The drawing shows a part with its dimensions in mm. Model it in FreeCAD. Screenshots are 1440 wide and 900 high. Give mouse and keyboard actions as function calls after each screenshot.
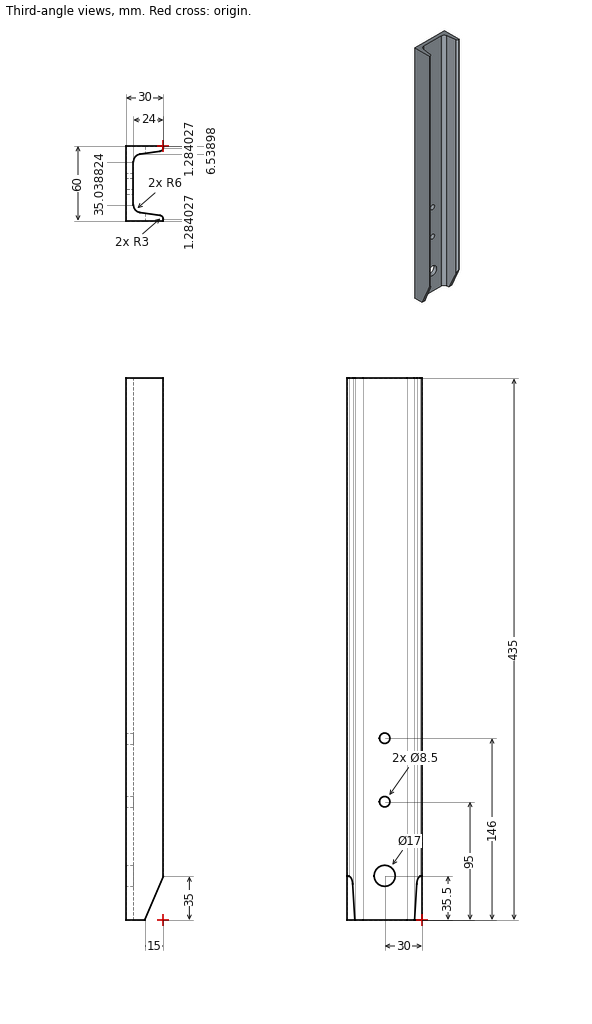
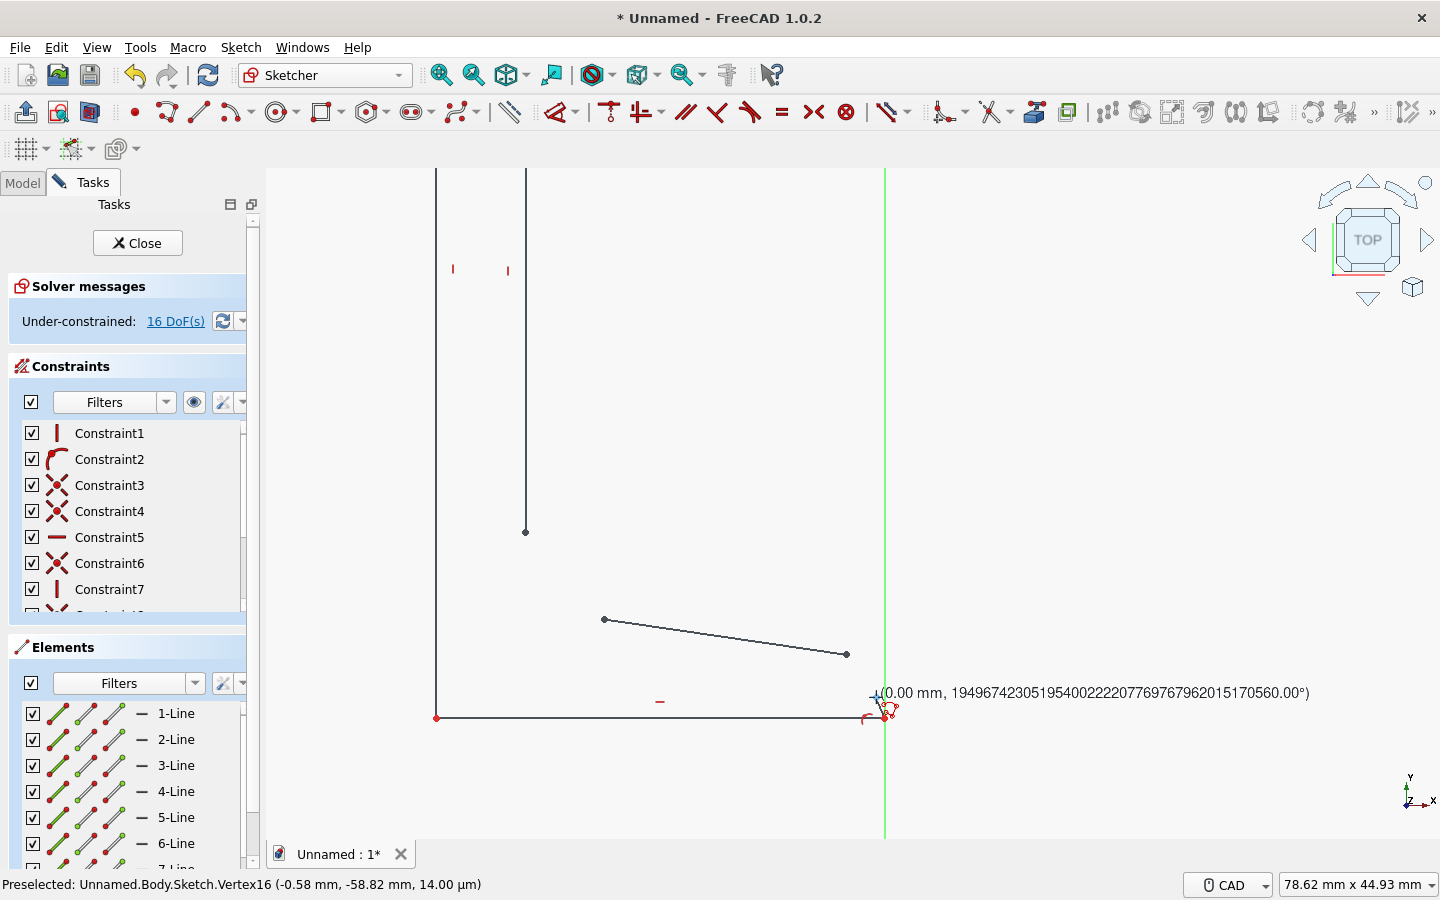
key(g)
key(3)
key(a)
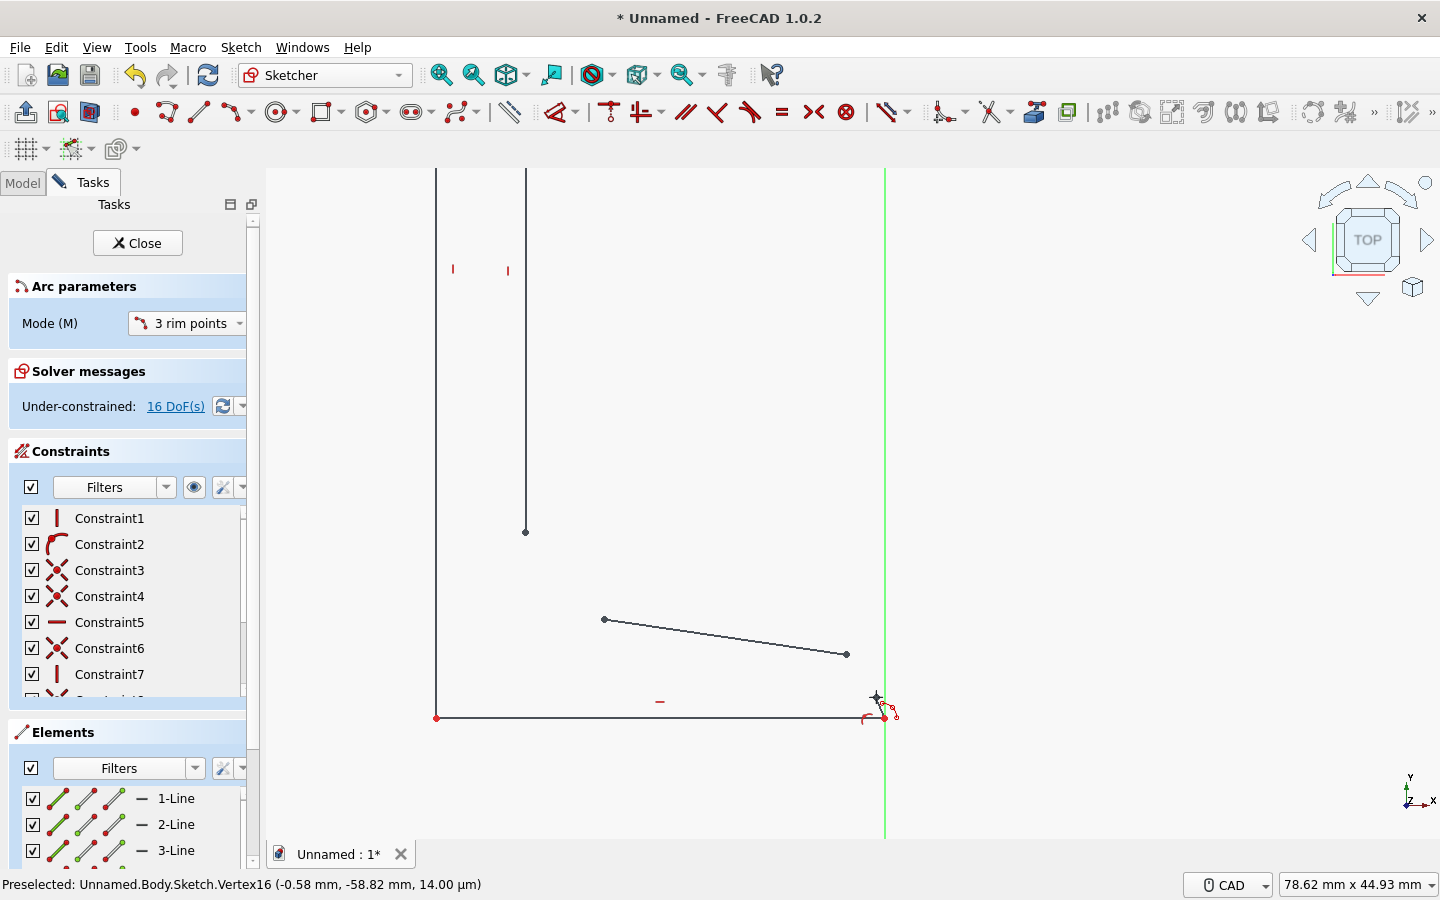
click(605, 619)
click(526, 533)
click(548, 588)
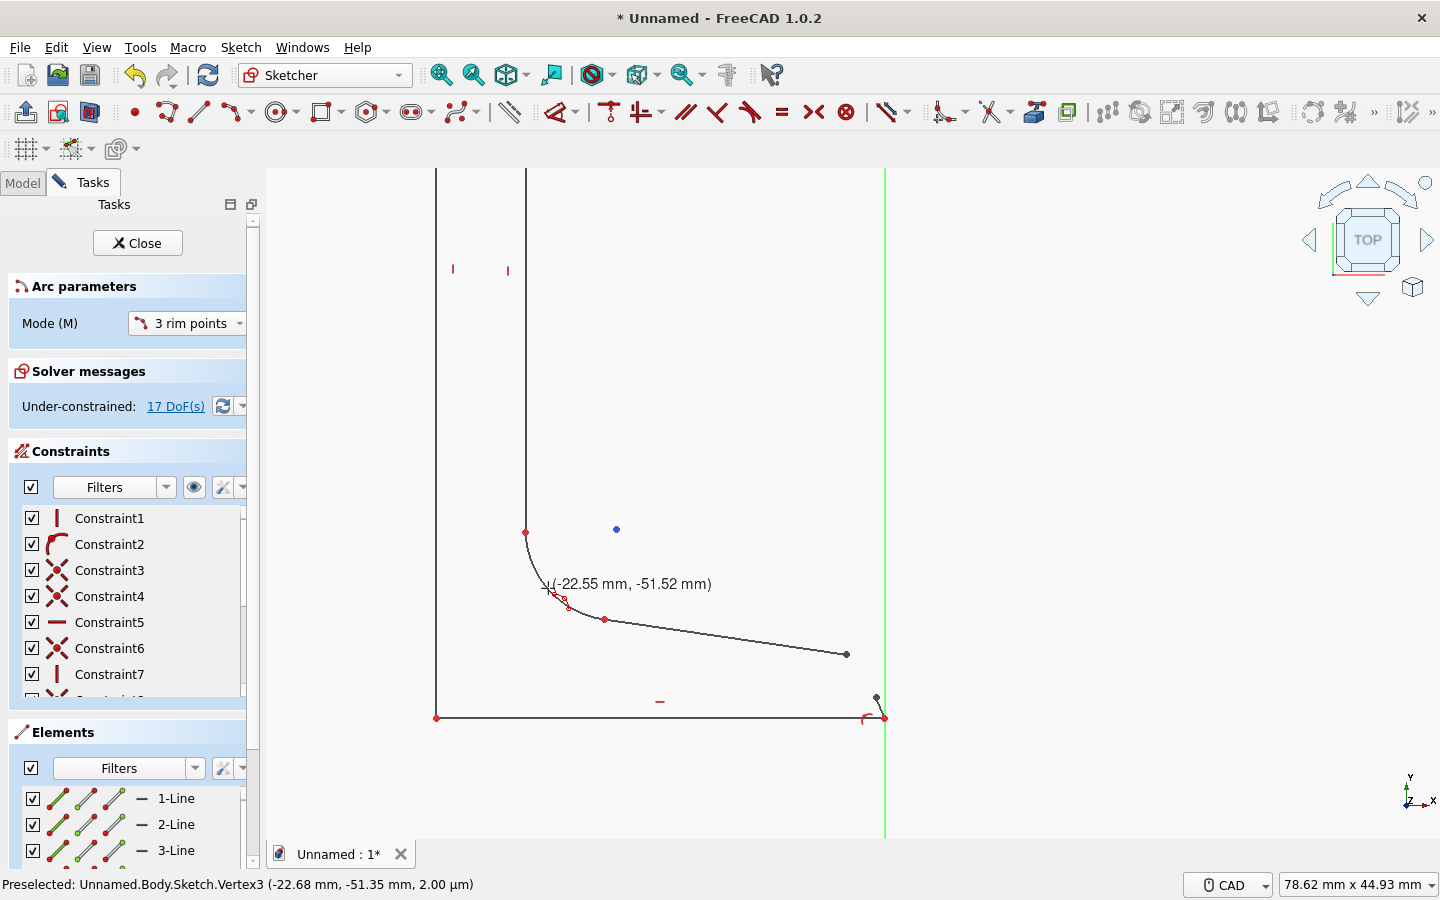
scroll(886, 696, down, 4)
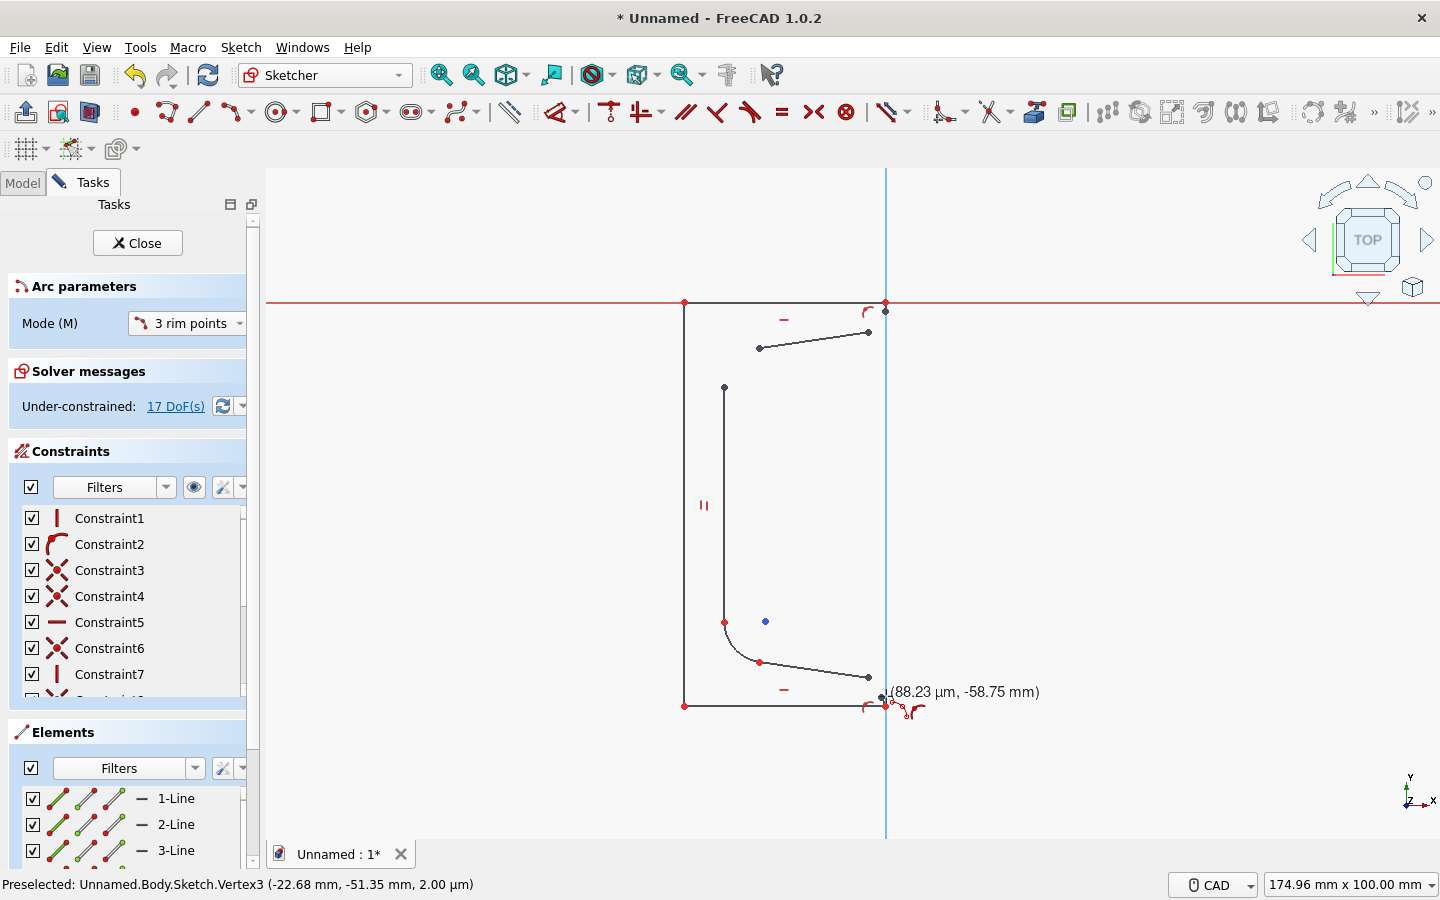
click(724, 387)
click(760, 348)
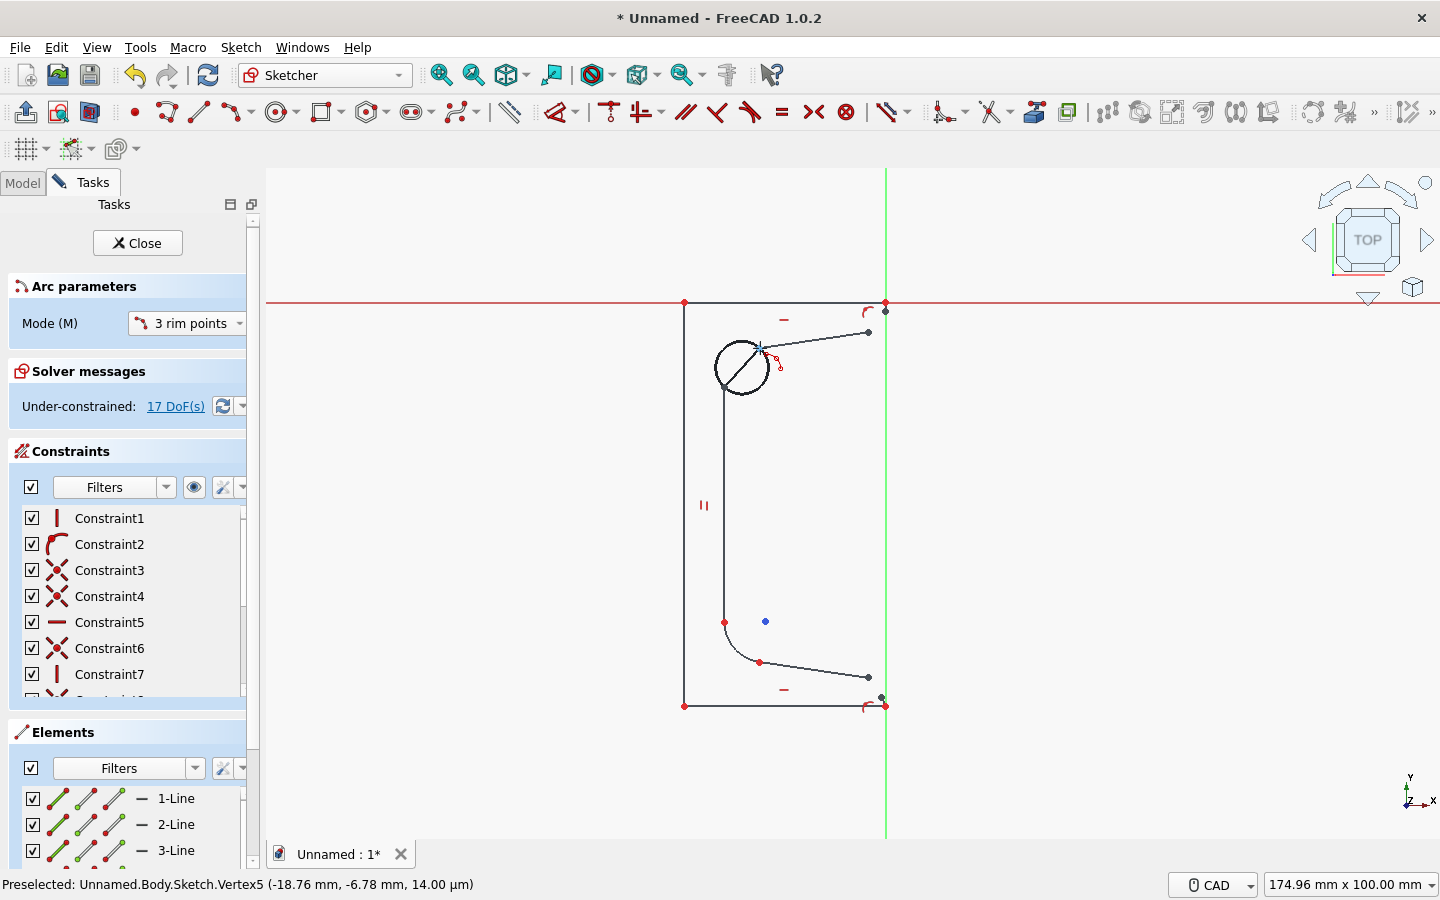
scroll(735, 360, up, 3)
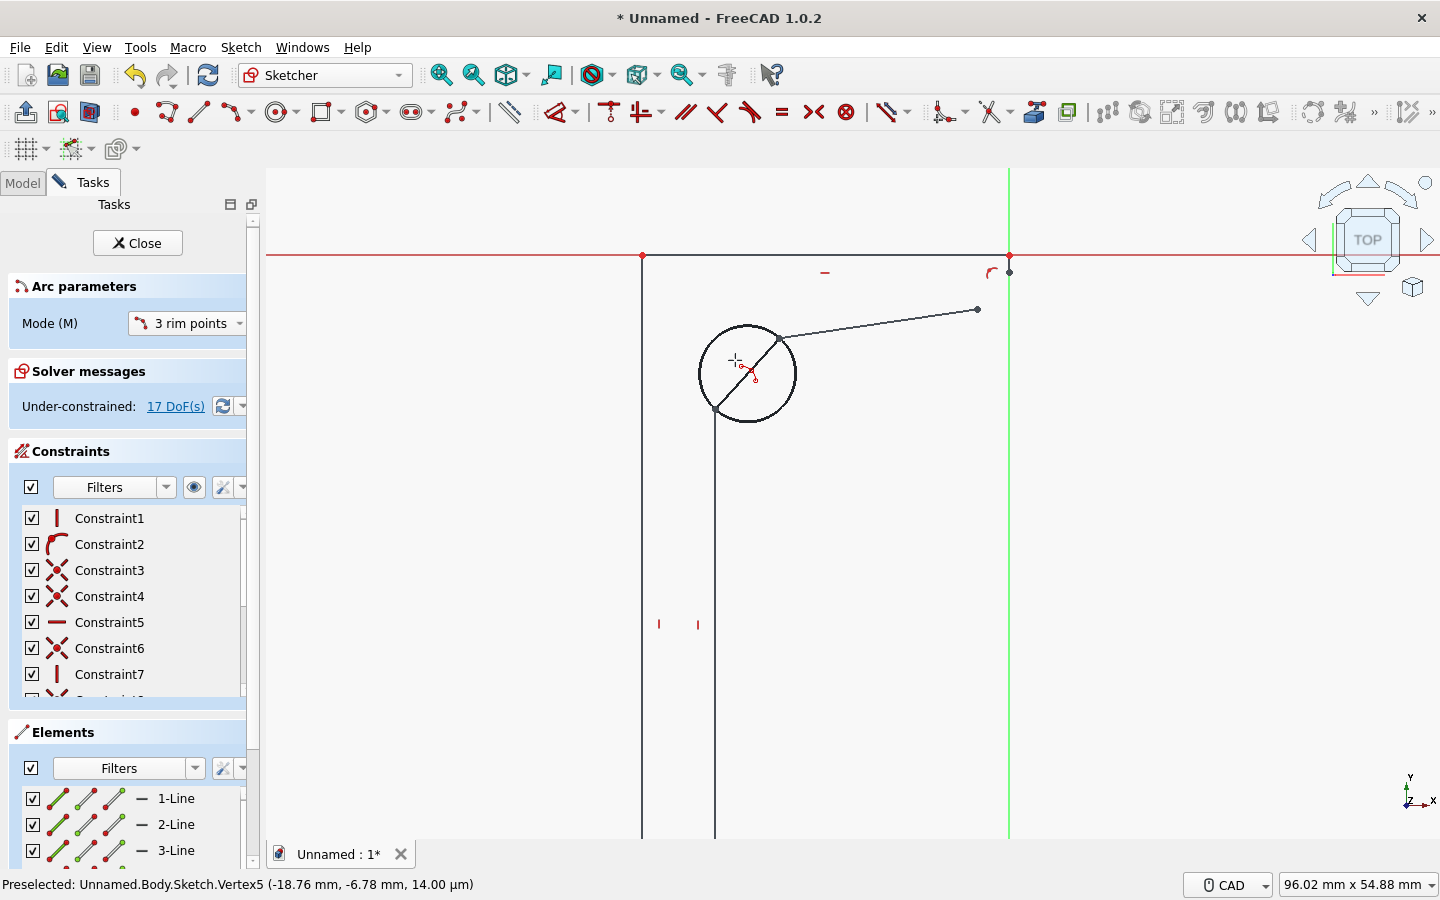
click(734, 360)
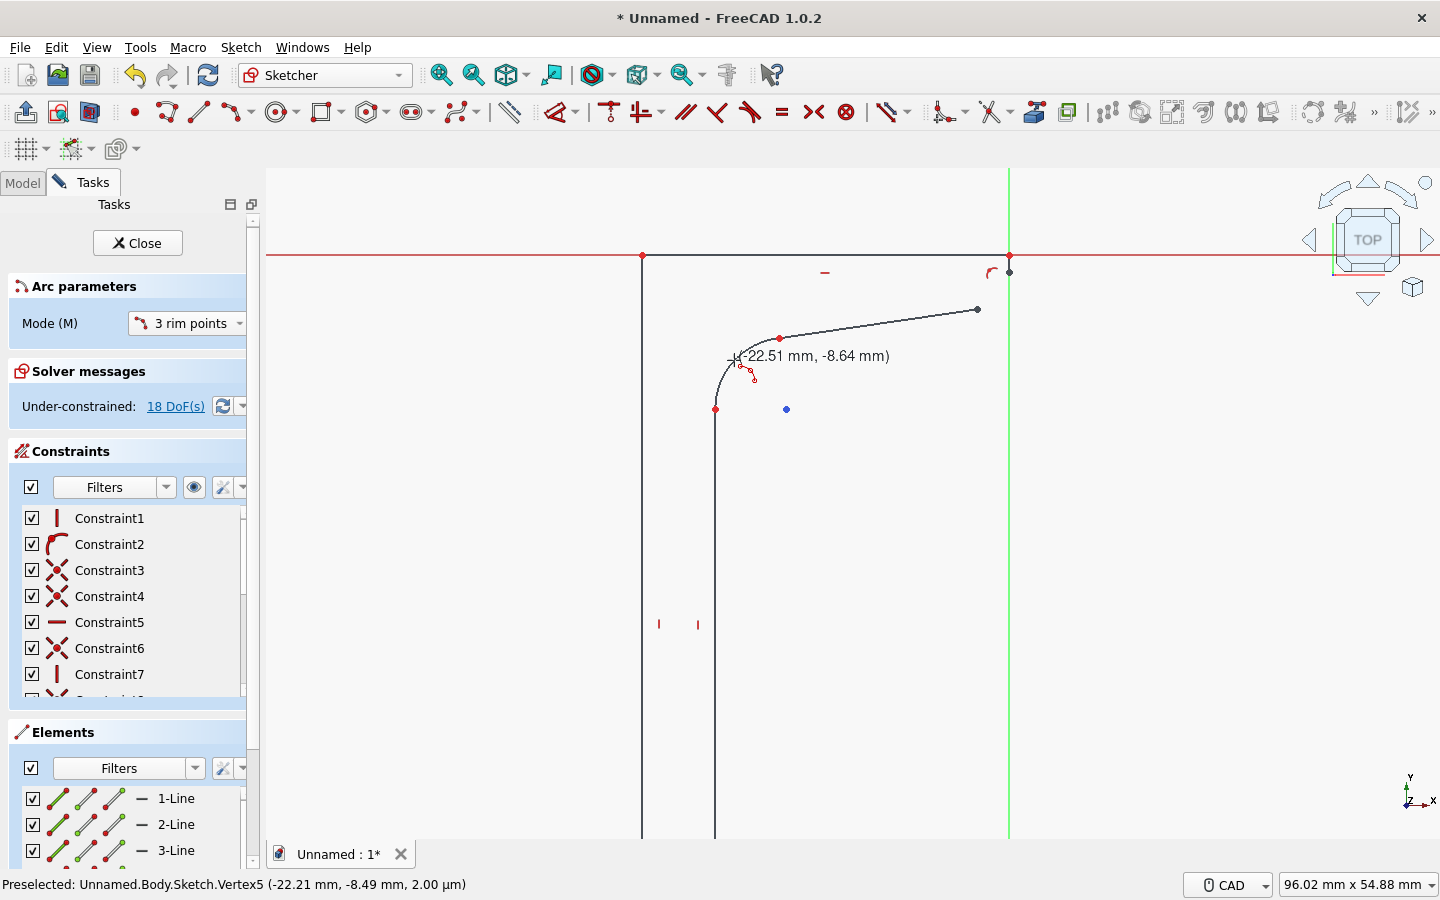
click(978, 309)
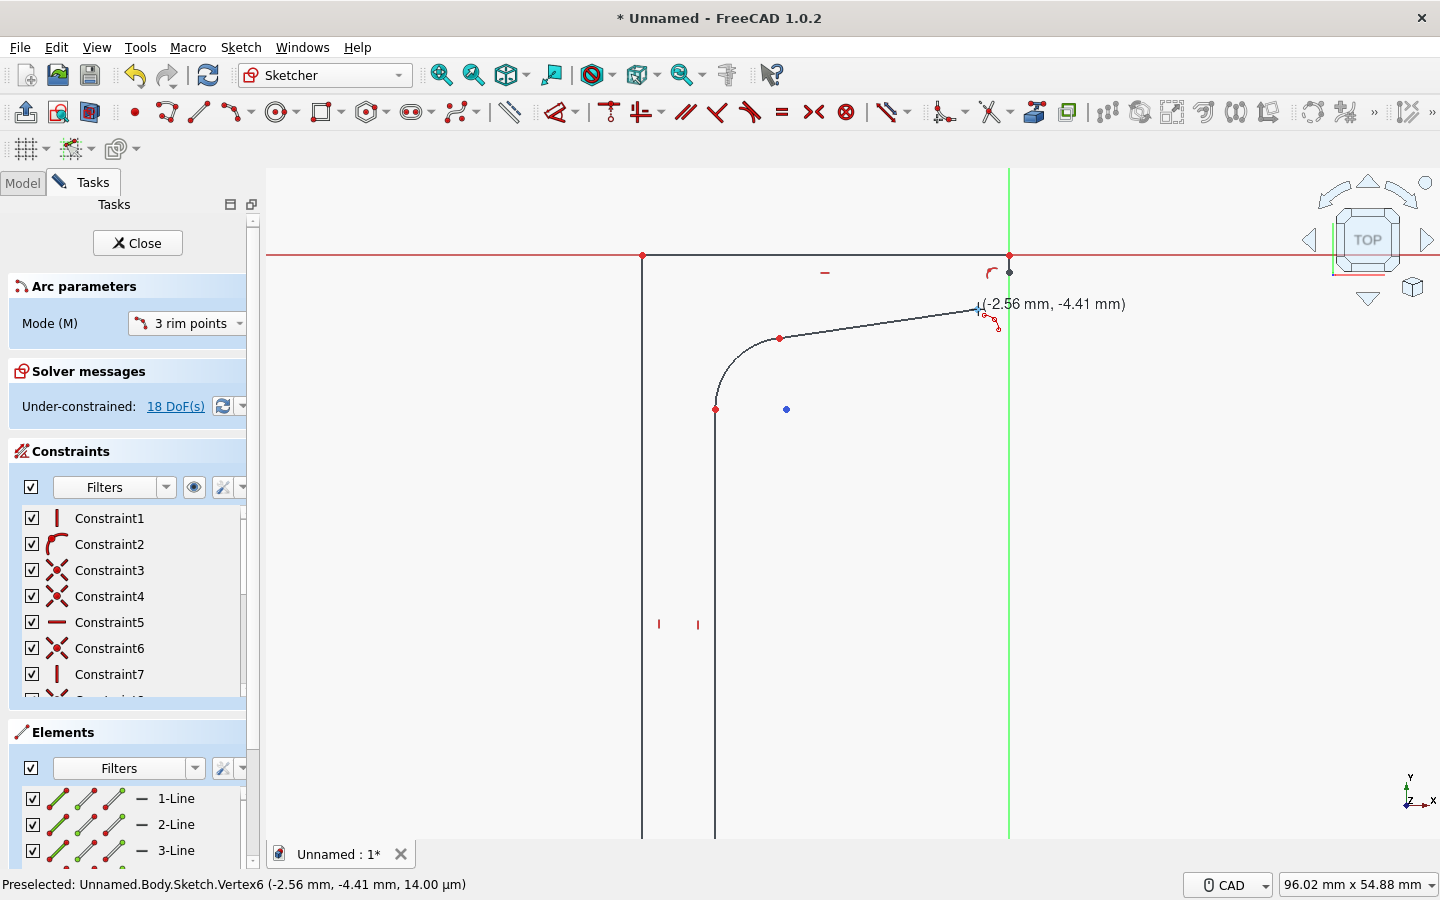
scroll(1009, 271, up, 4)